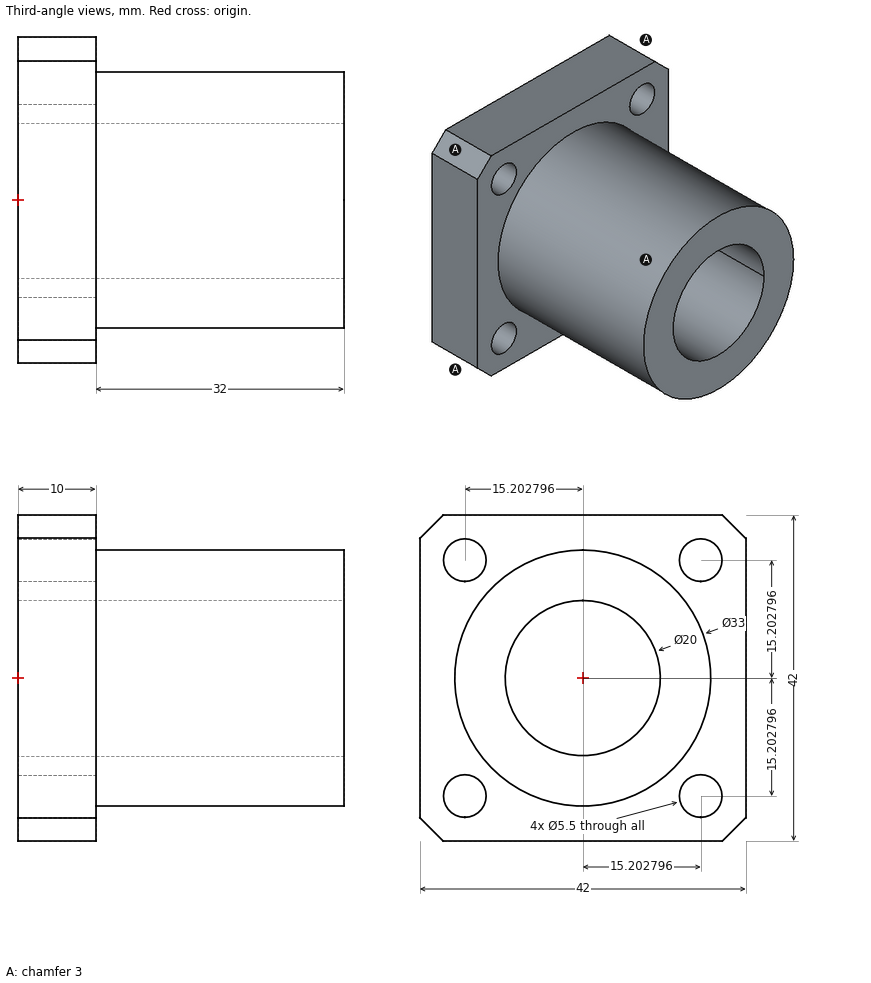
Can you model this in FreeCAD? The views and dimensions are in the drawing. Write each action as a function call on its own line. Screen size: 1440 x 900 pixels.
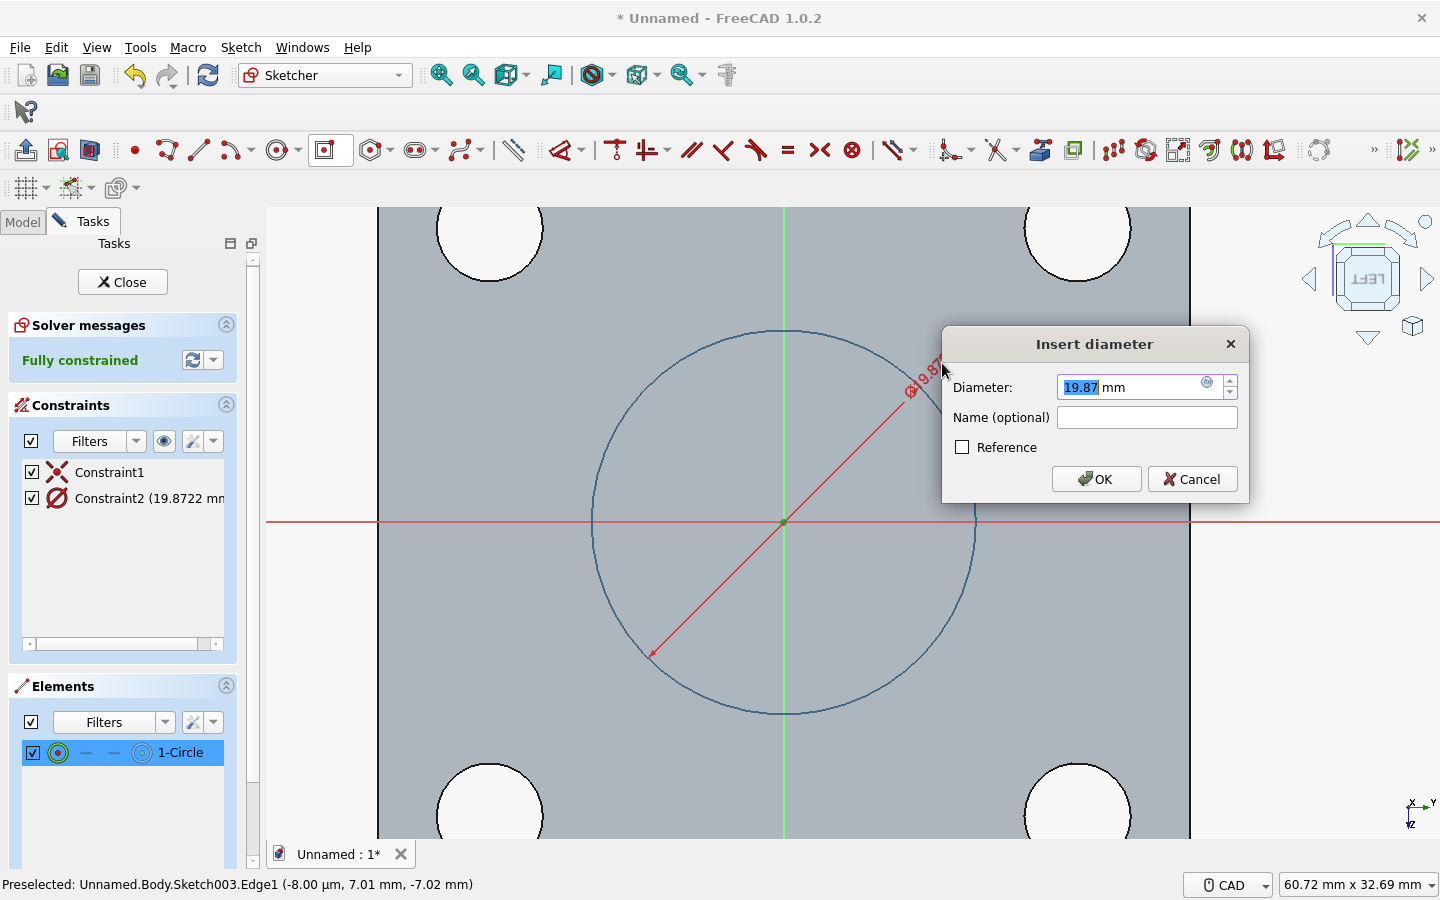
text(20)
key(Return)
key(Escape)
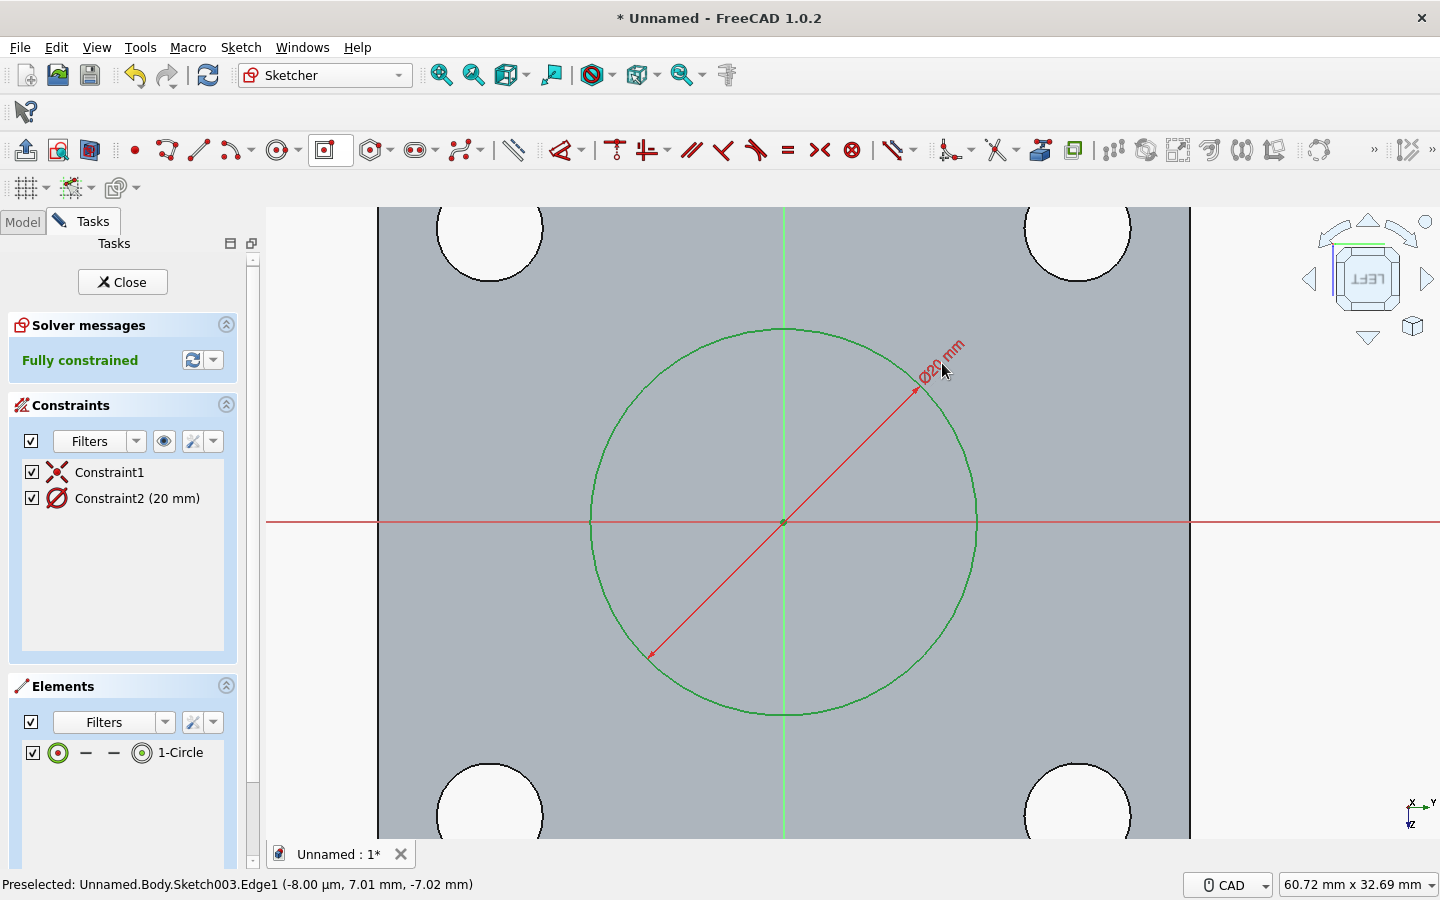
click(123, 282)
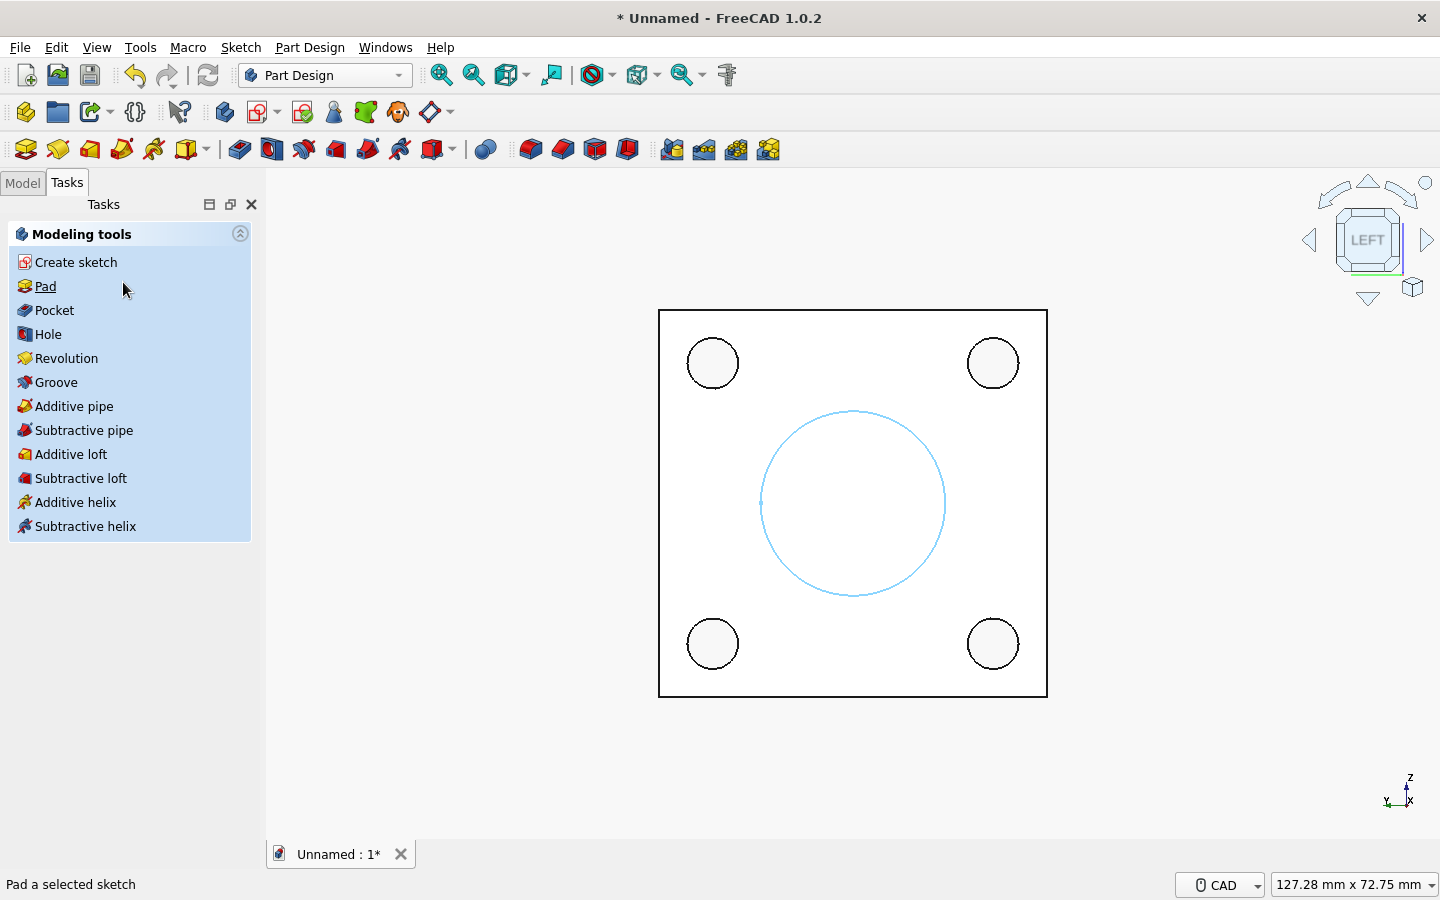
click(240, 150)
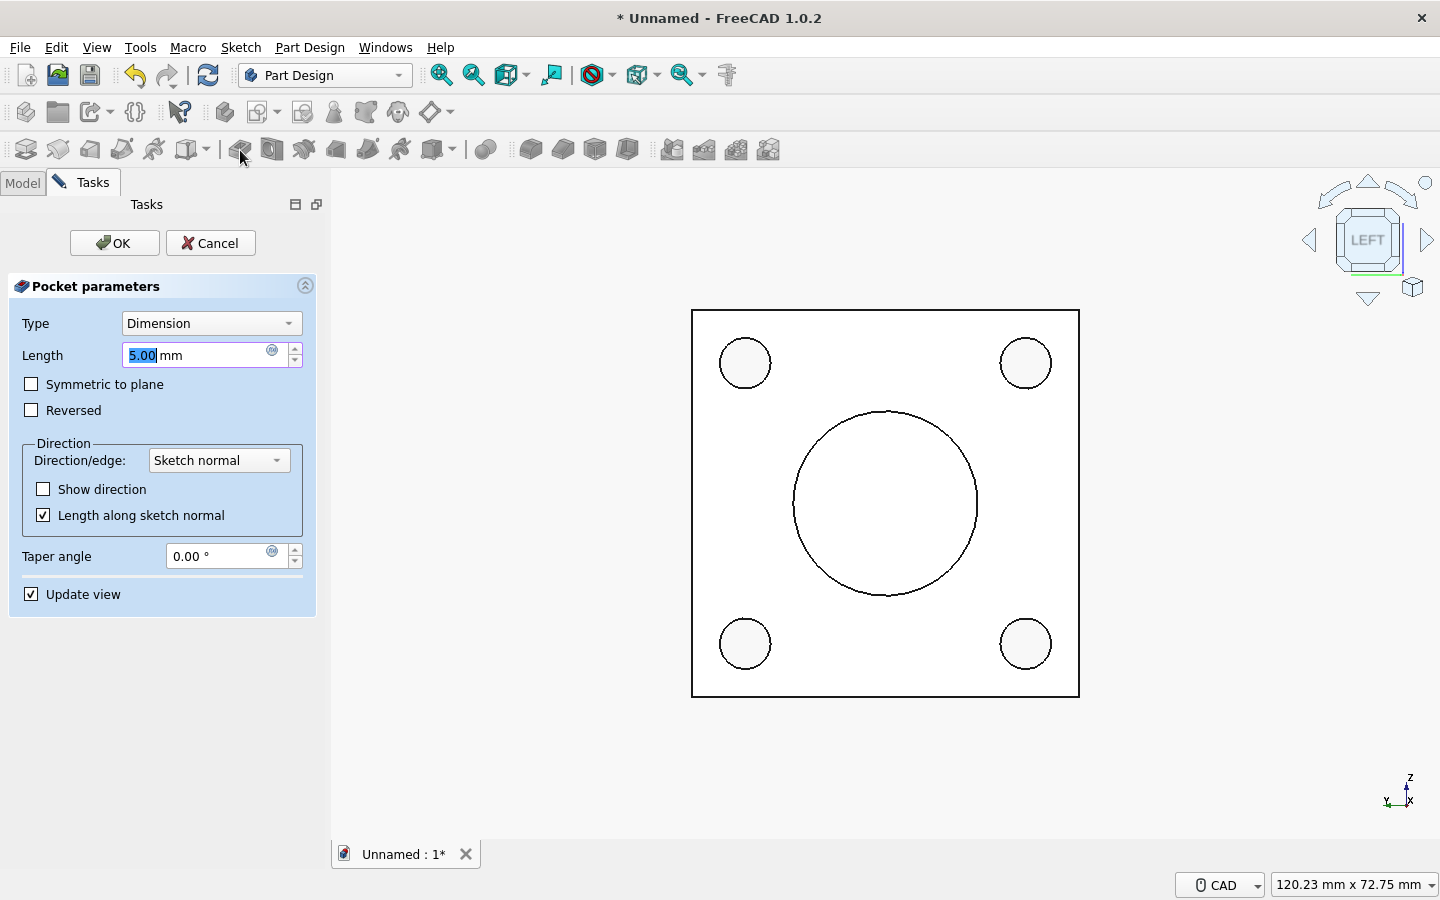
click(212, 324)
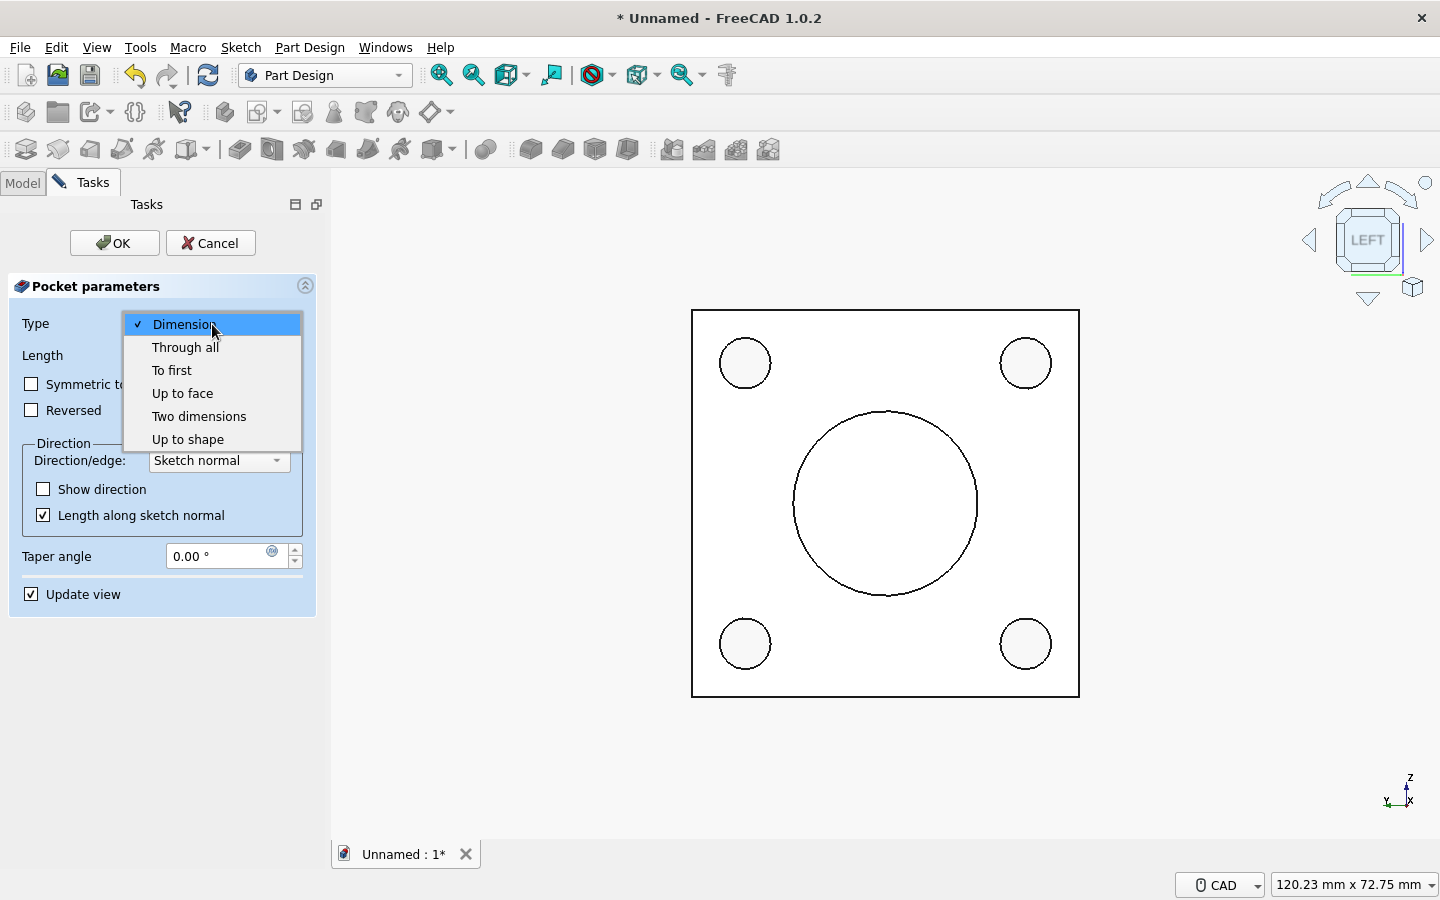
click(212, 348)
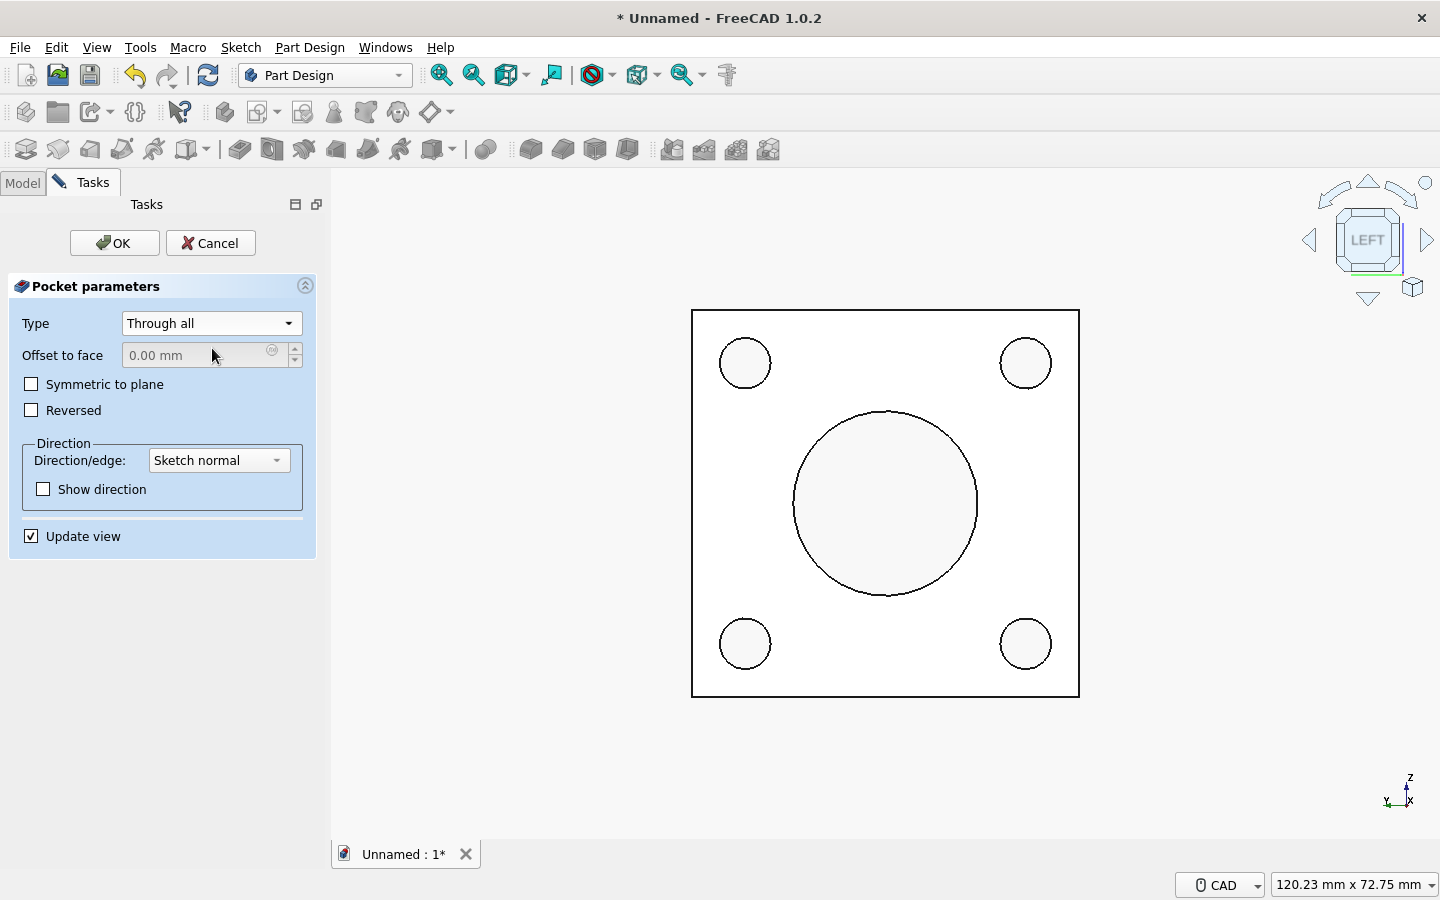
click(115, 243)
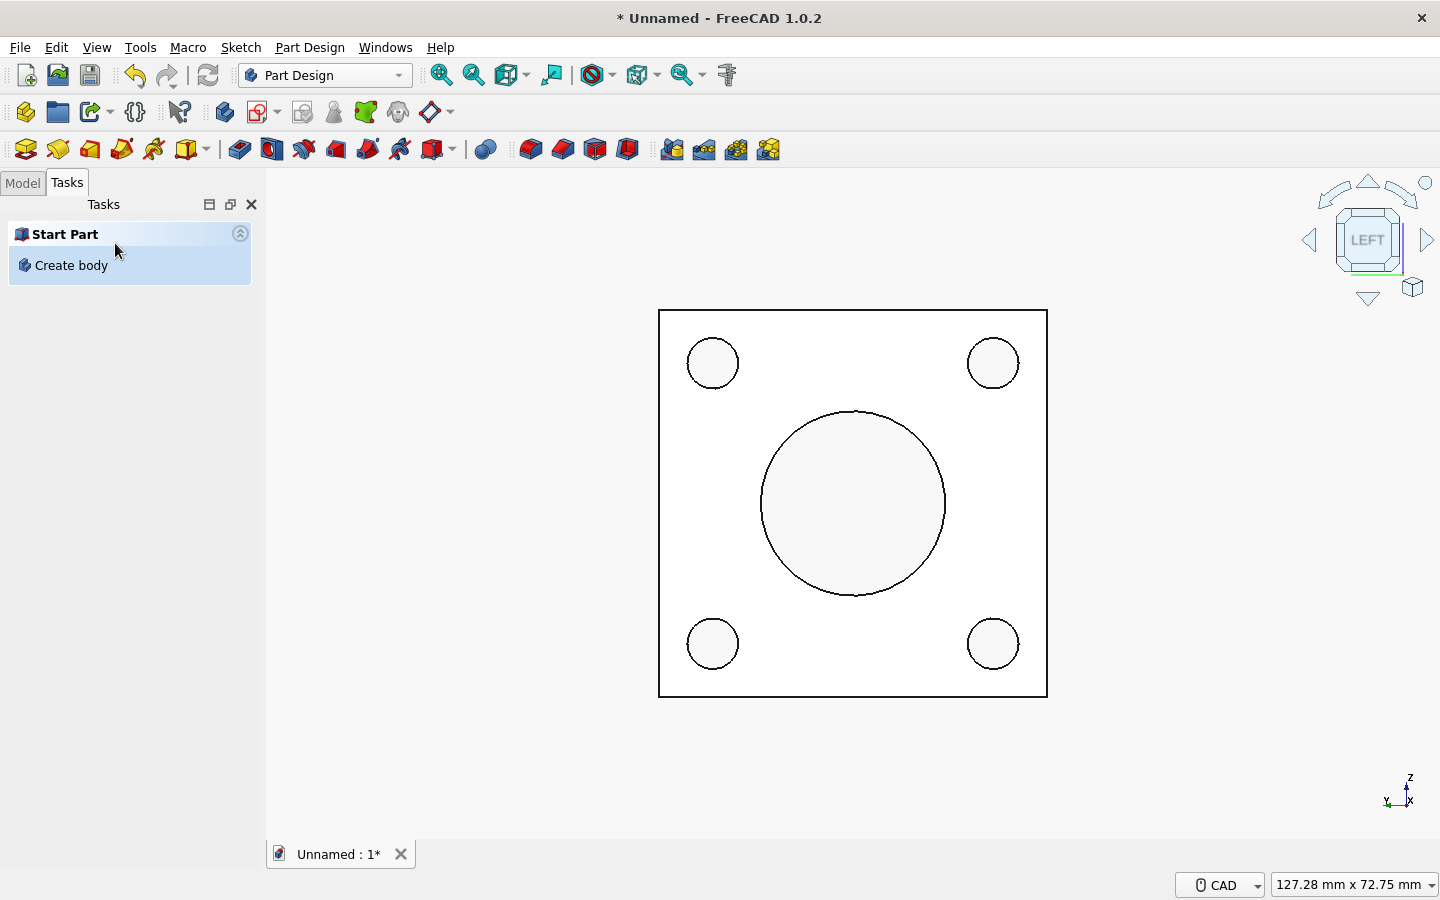
key(0)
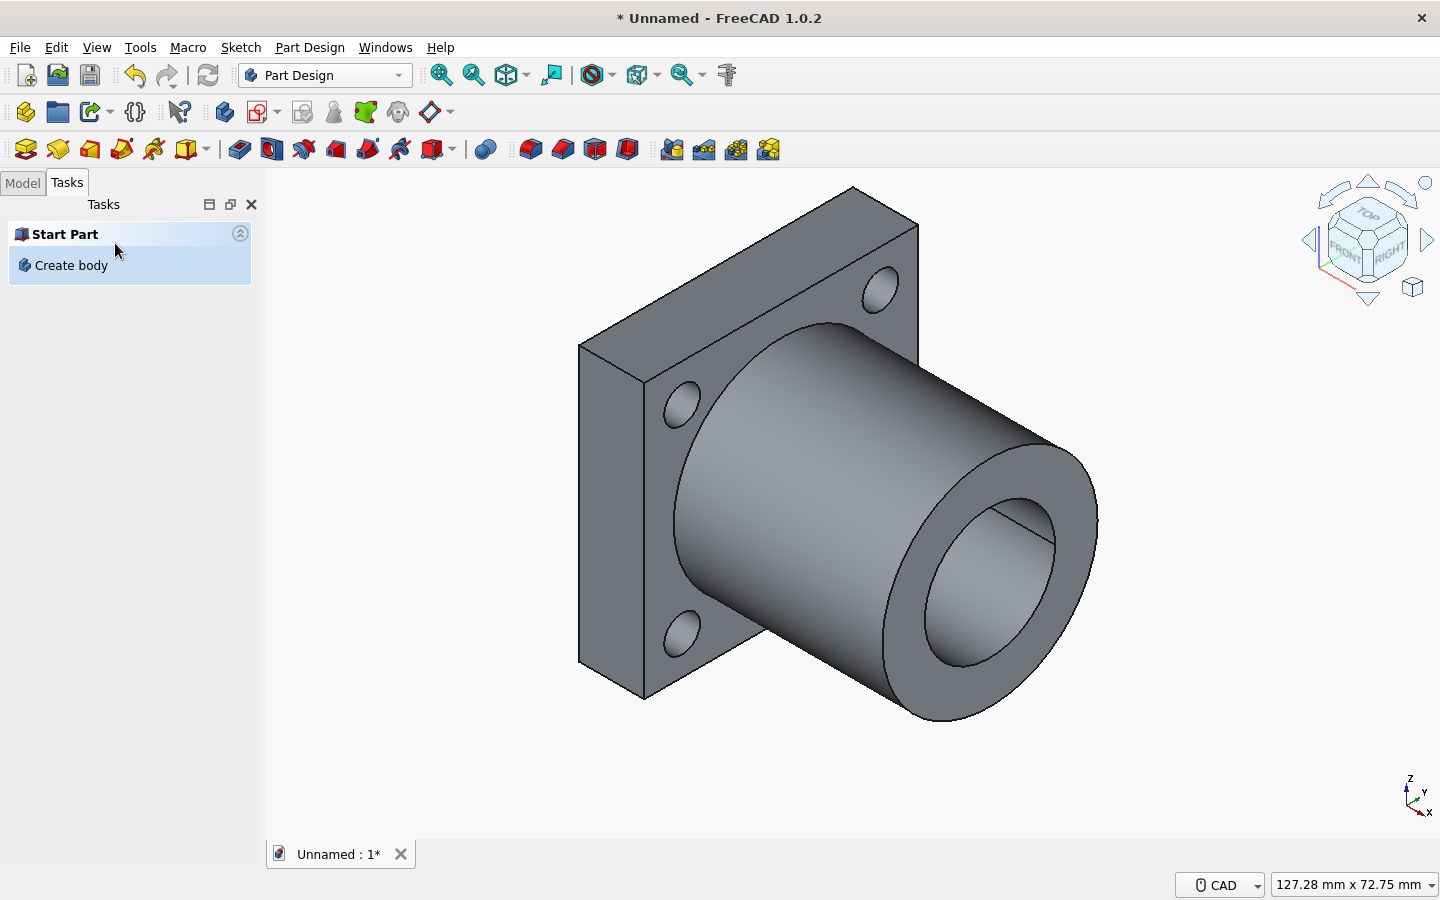
click(612, 363)